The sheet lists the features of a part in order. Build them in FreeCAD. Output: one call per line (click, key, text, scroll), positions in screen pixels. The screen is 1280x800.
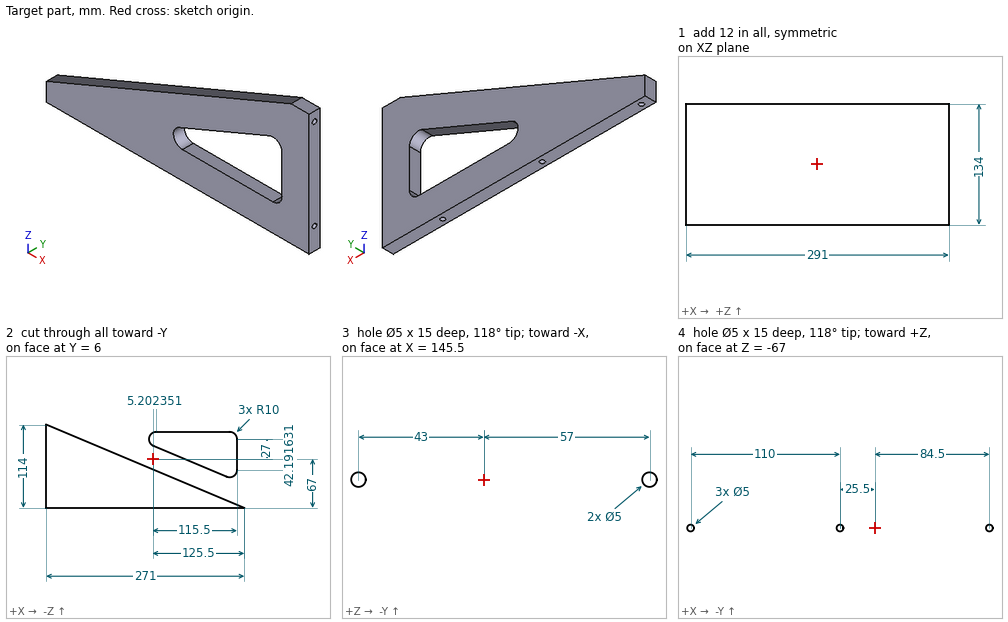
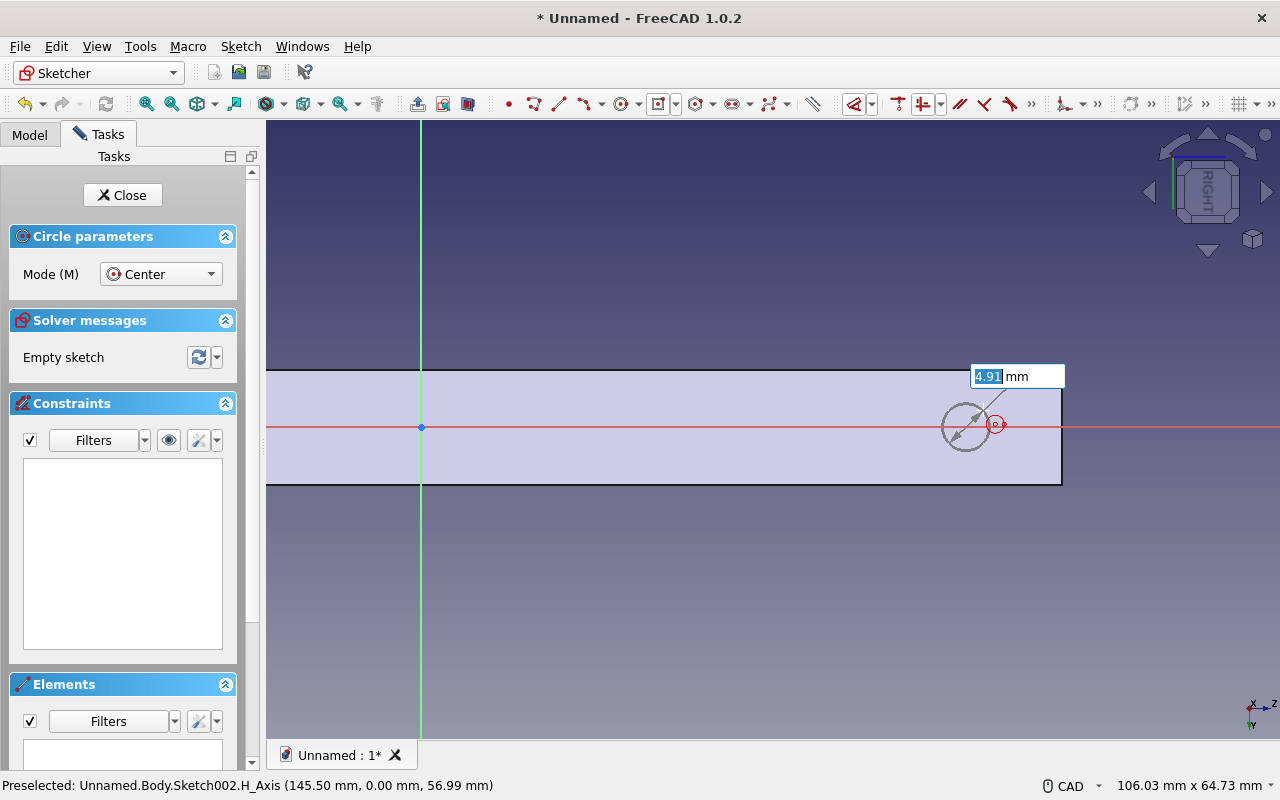
text(5)
key(Return)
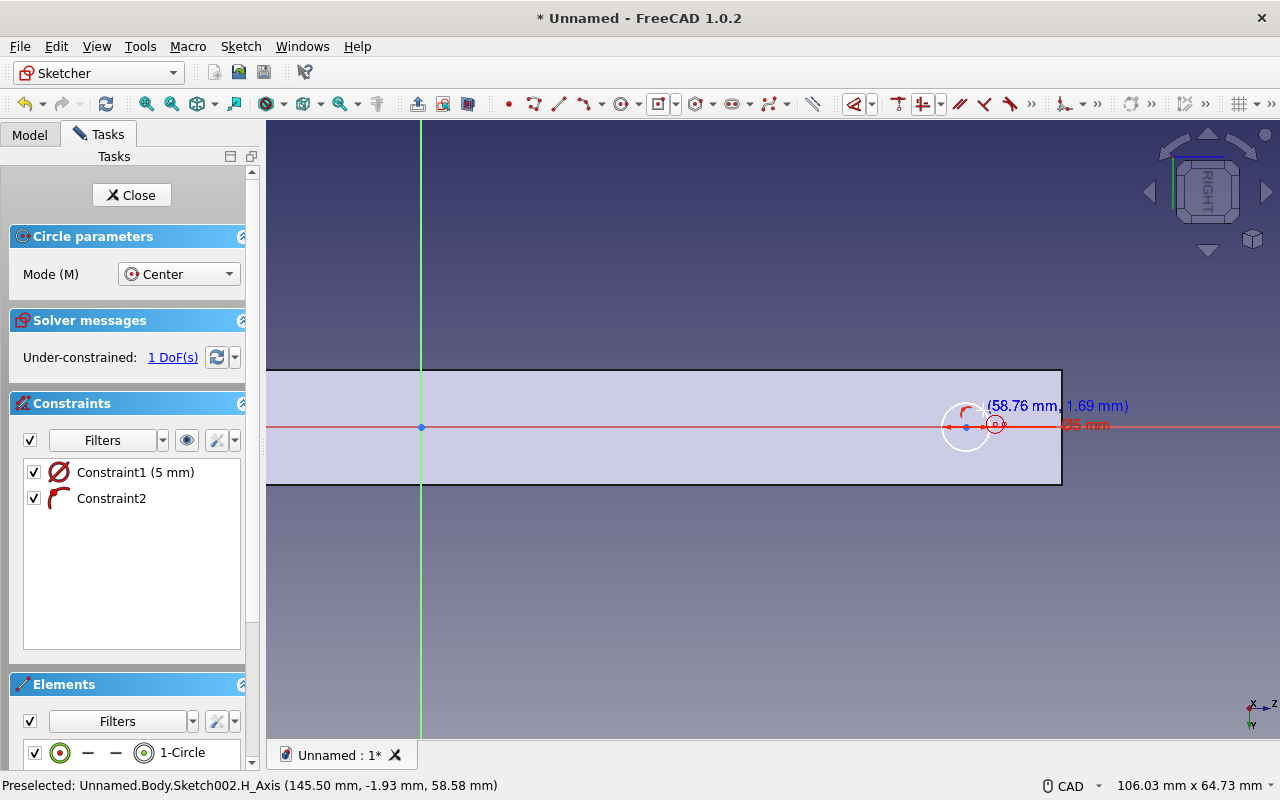
scroll(968, 432, down, 3)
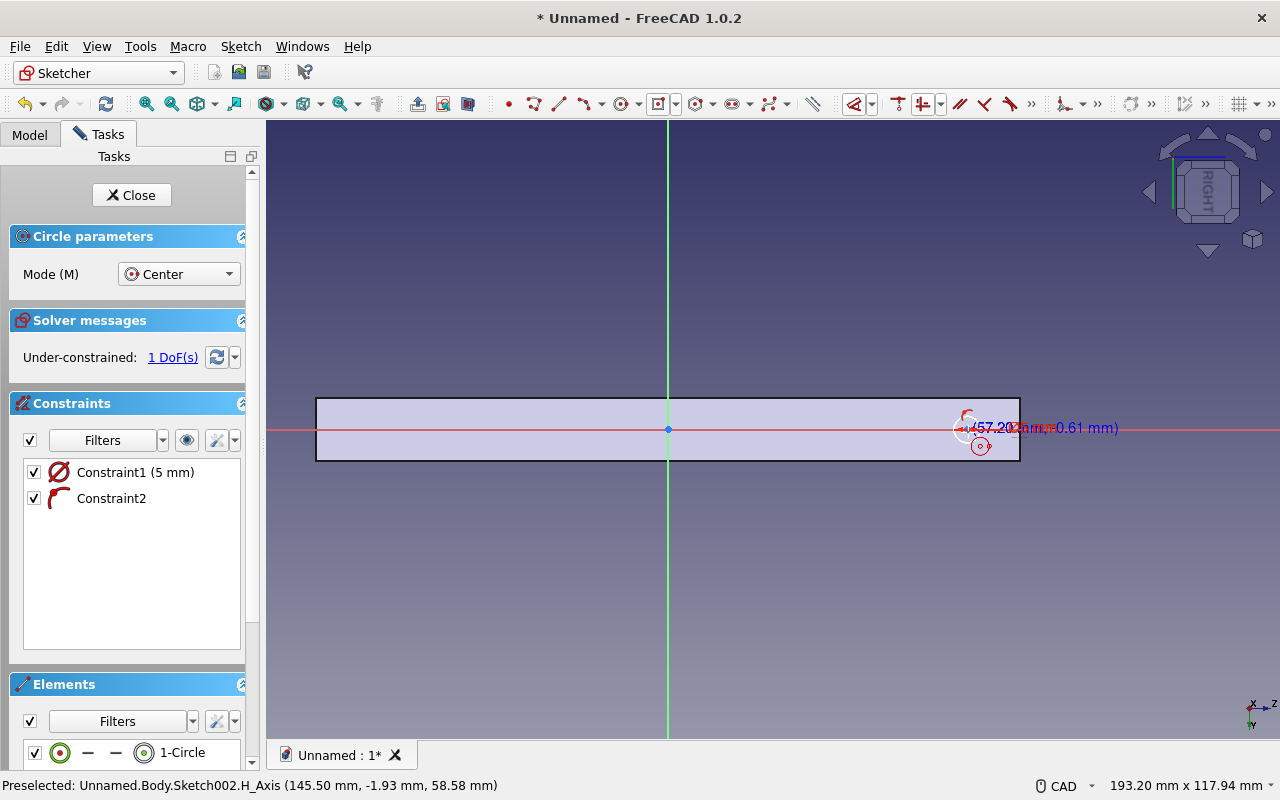
scroll(442, 430, up, 3)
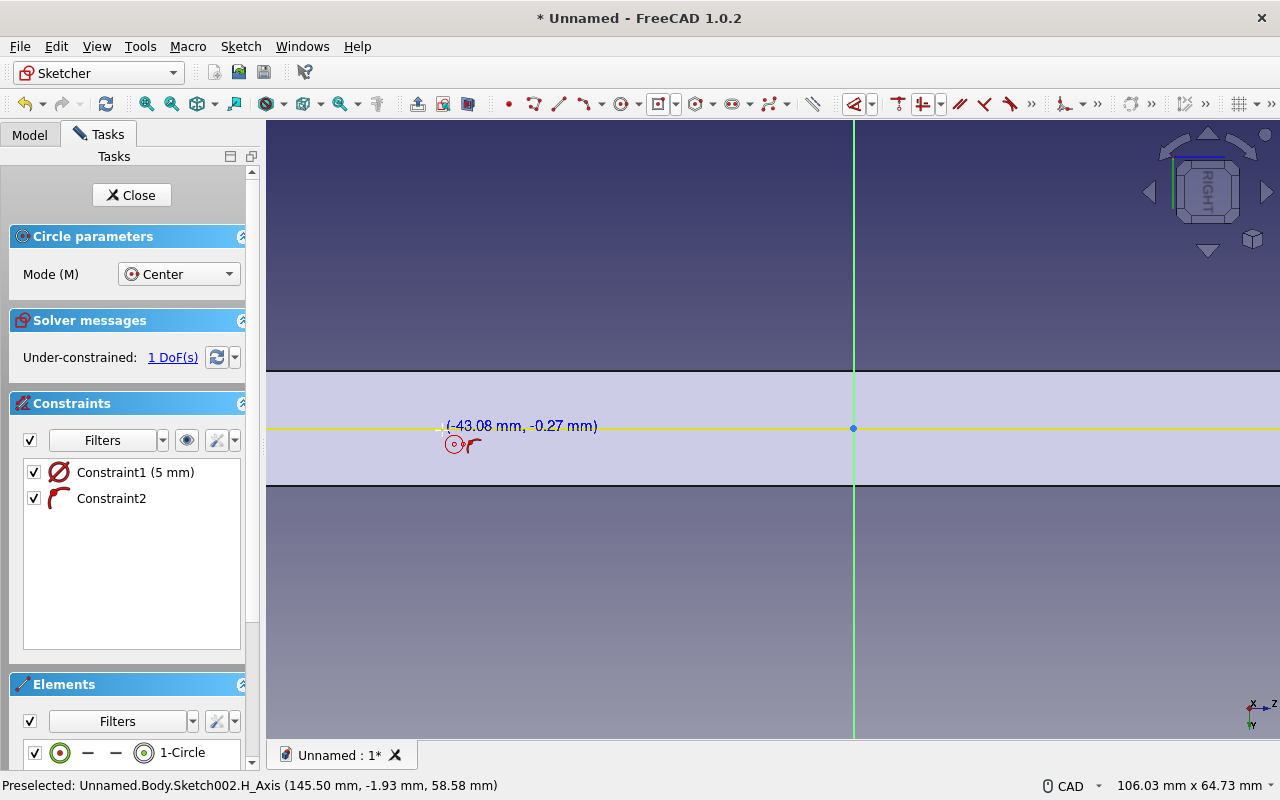
click(443, 429)
move(460, 412)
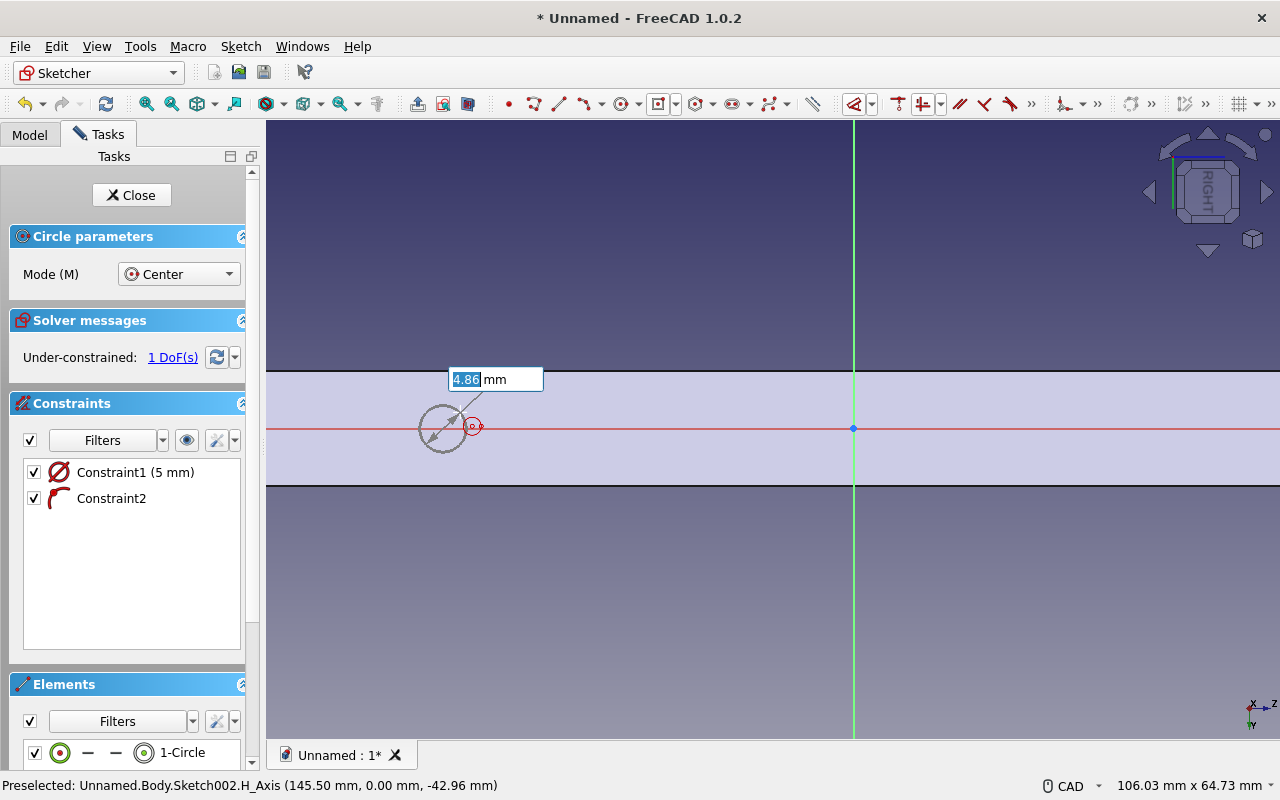
text(5)
key(Return)
key(Escape)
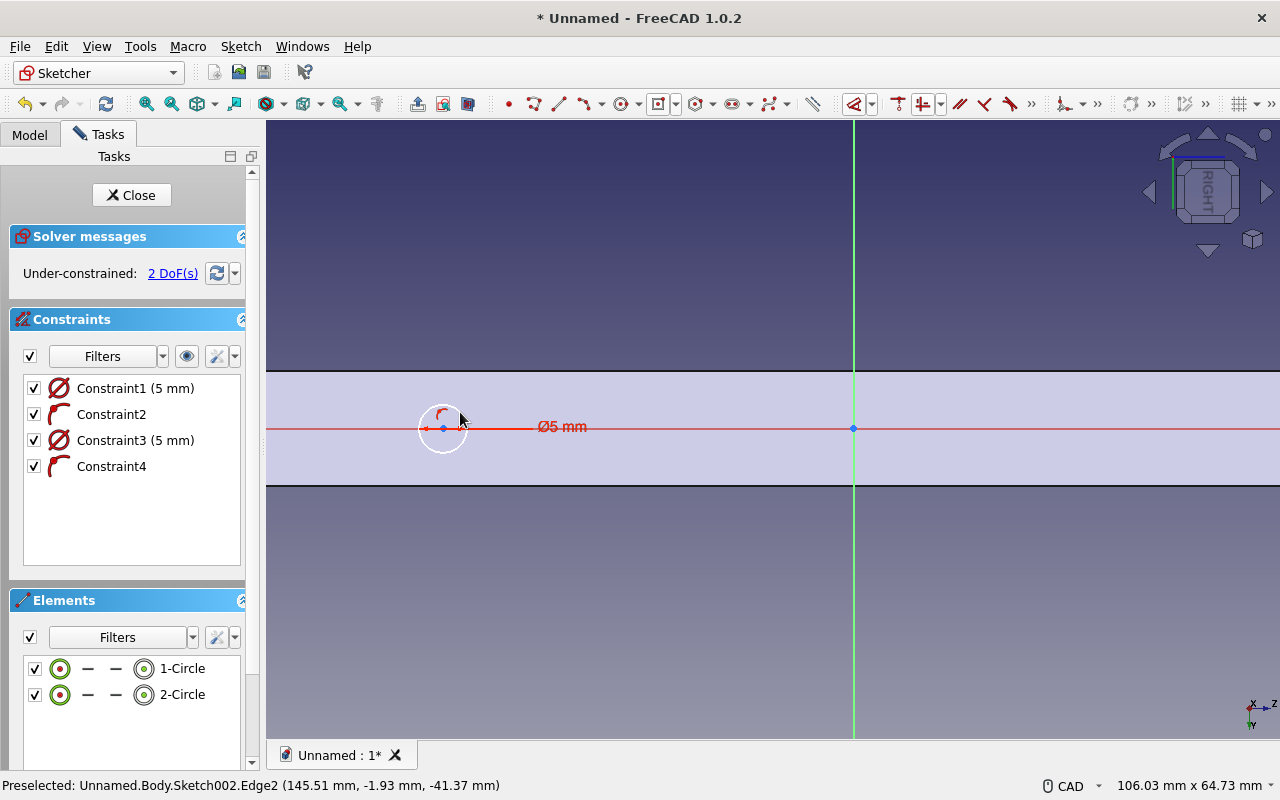
click(854, 104)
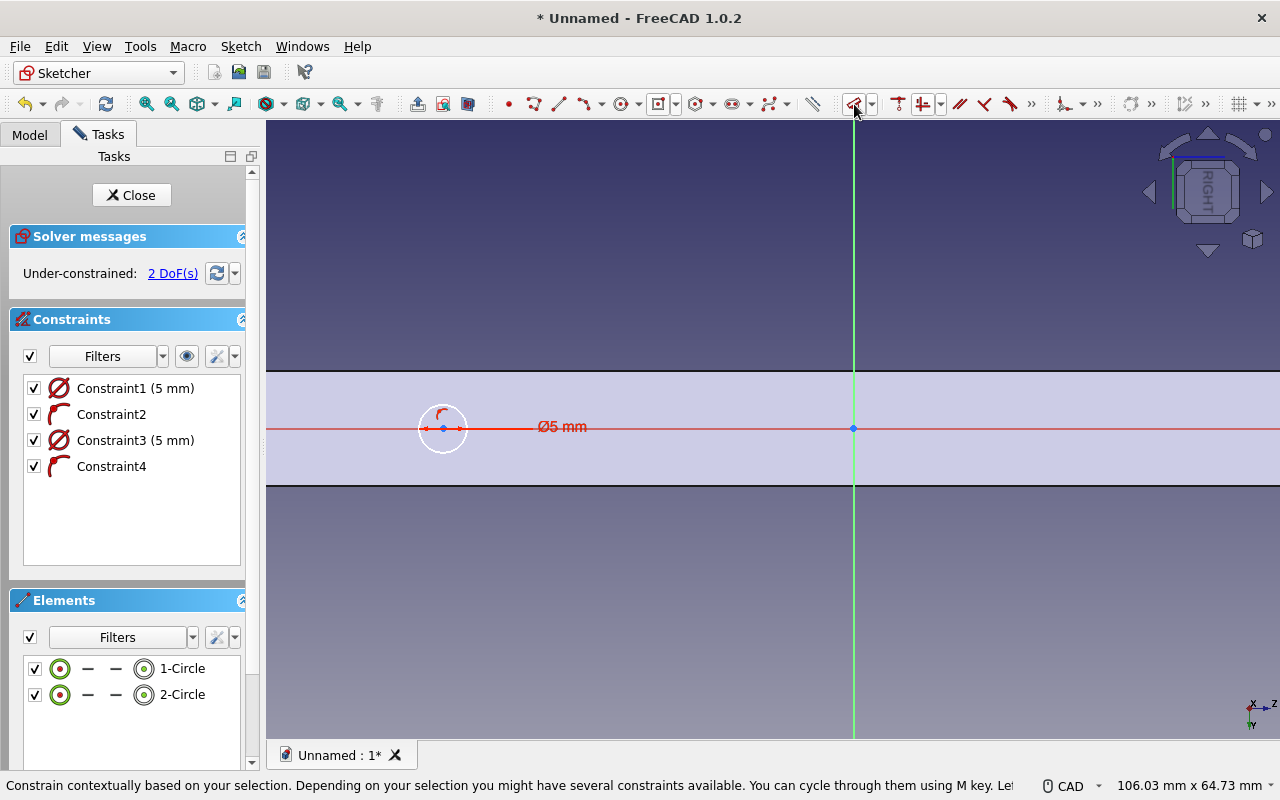
scroll(441, 430, down, 3)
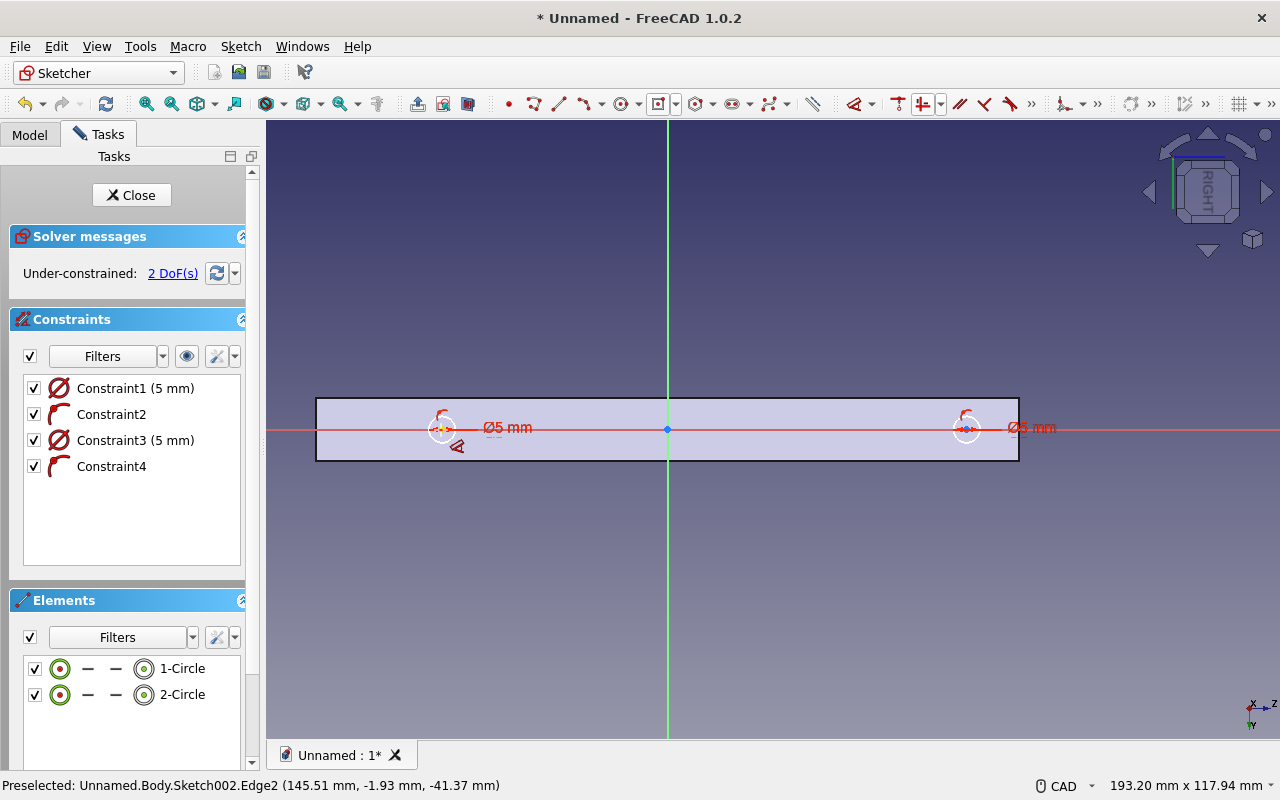
click(967, 430)
click(817, 464)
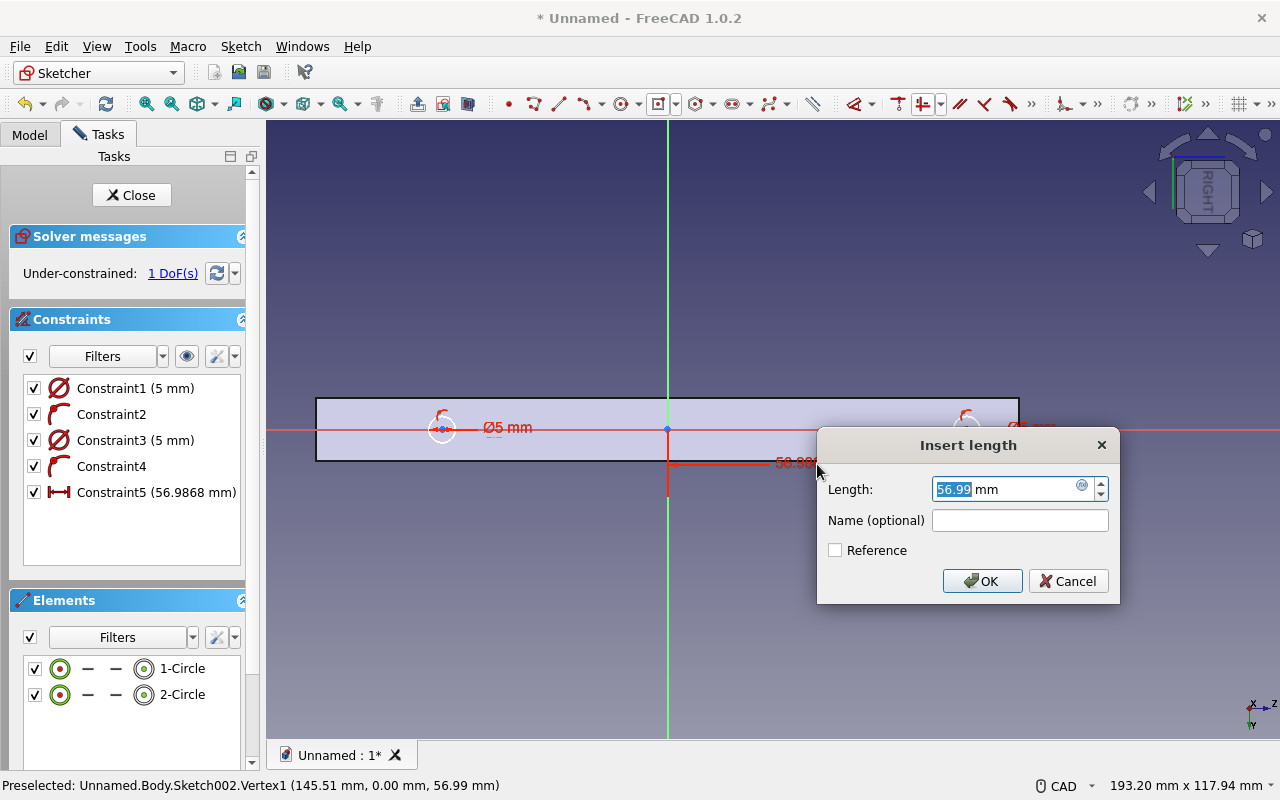
text(57)
key(Return)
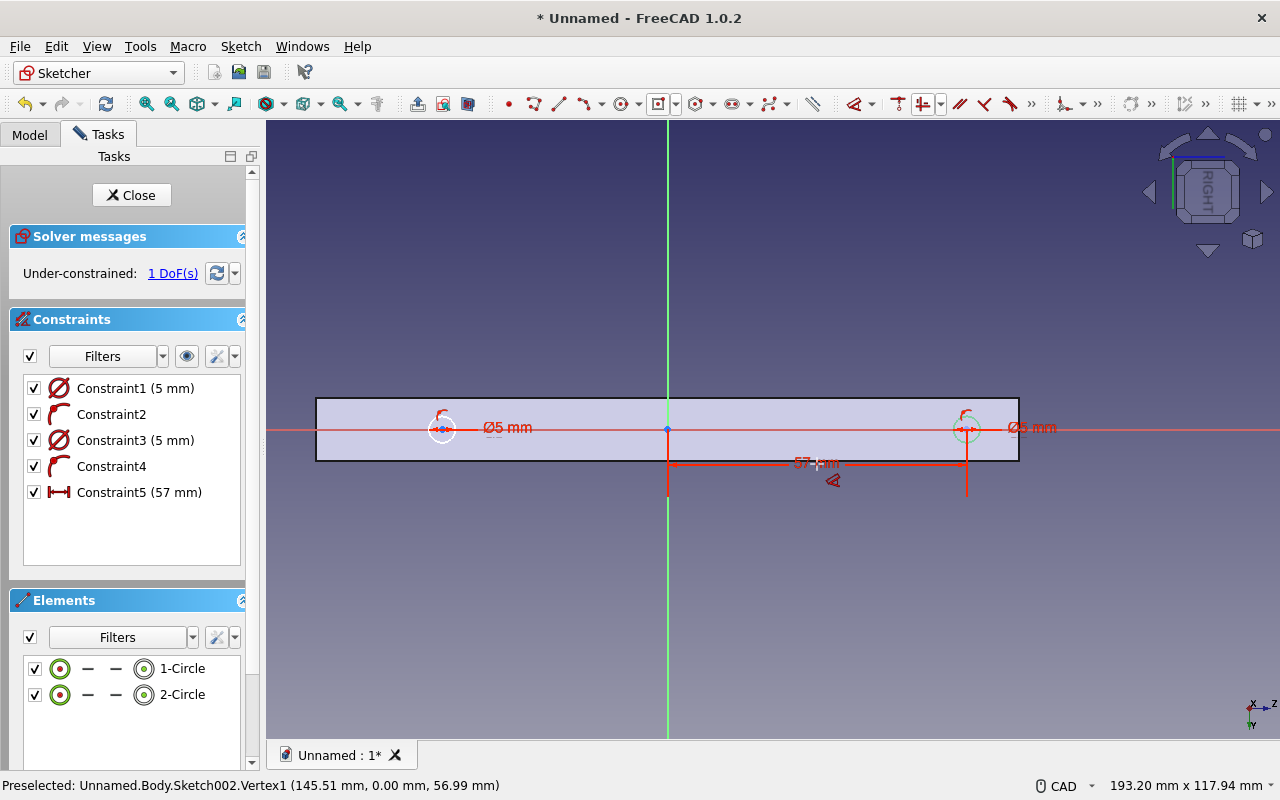
click(442, 430)
click(555, 464)